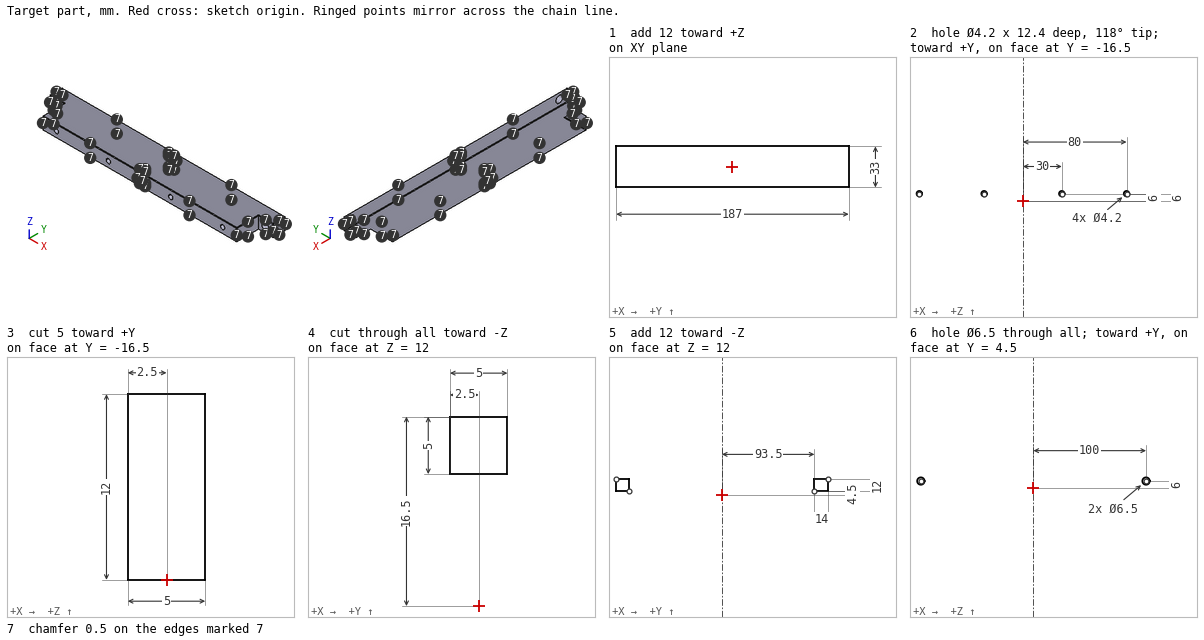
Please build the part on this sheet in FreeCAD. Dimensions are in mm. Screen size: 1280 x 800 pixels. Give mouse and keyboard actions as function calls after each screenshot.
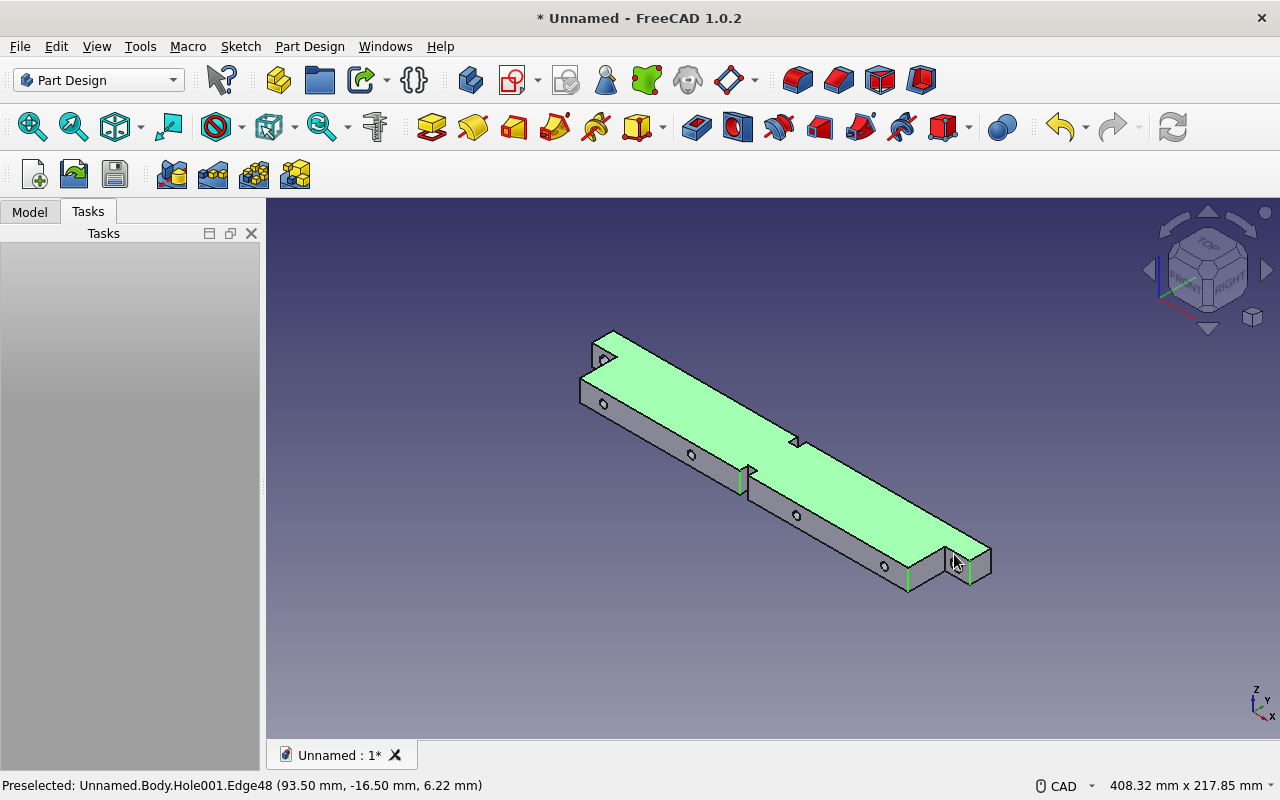
key(2)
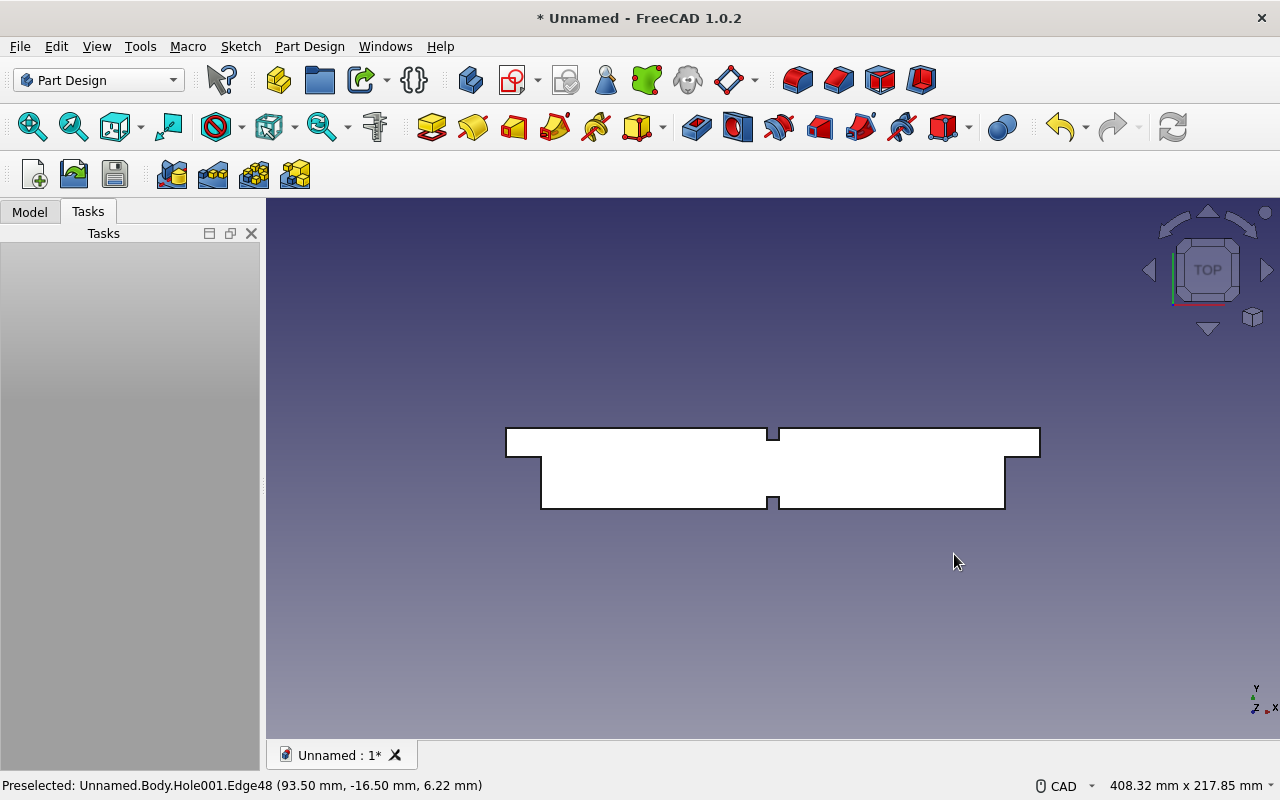
key(1)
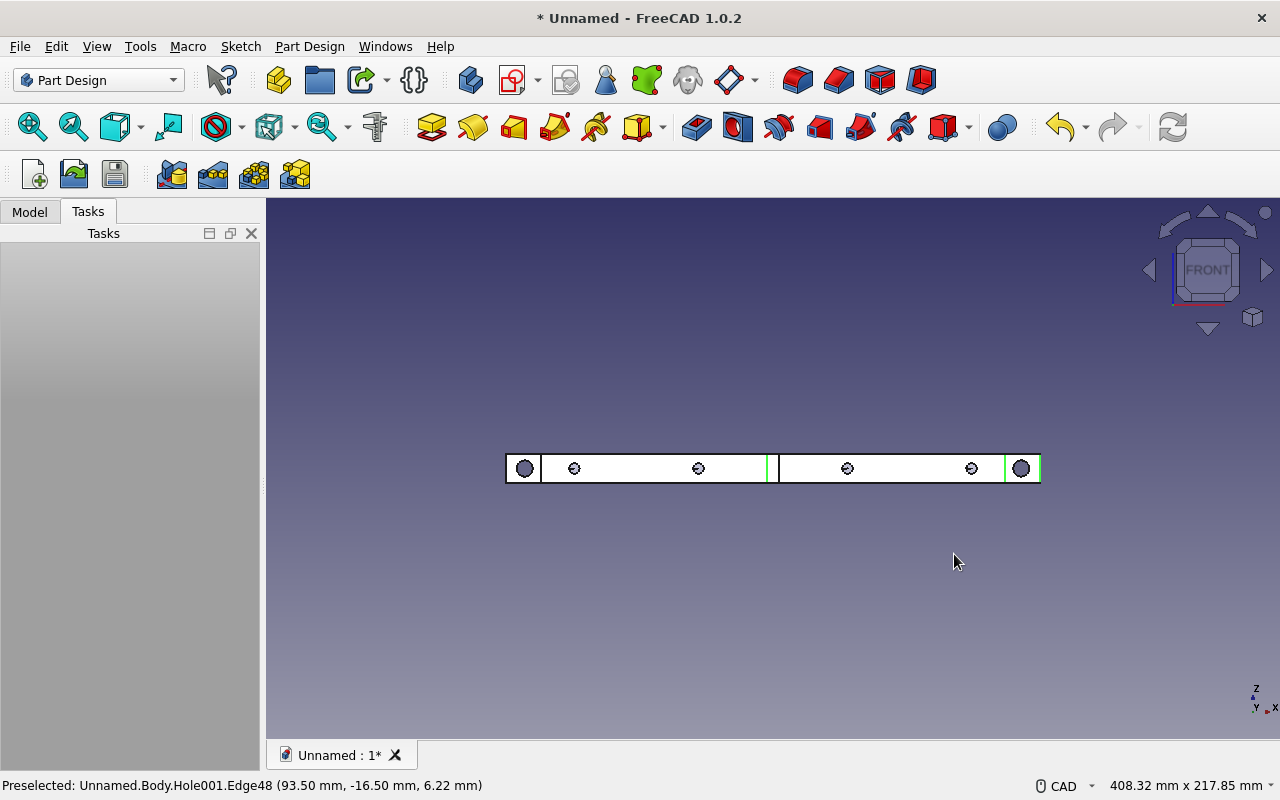
click(779, 467, ctrl)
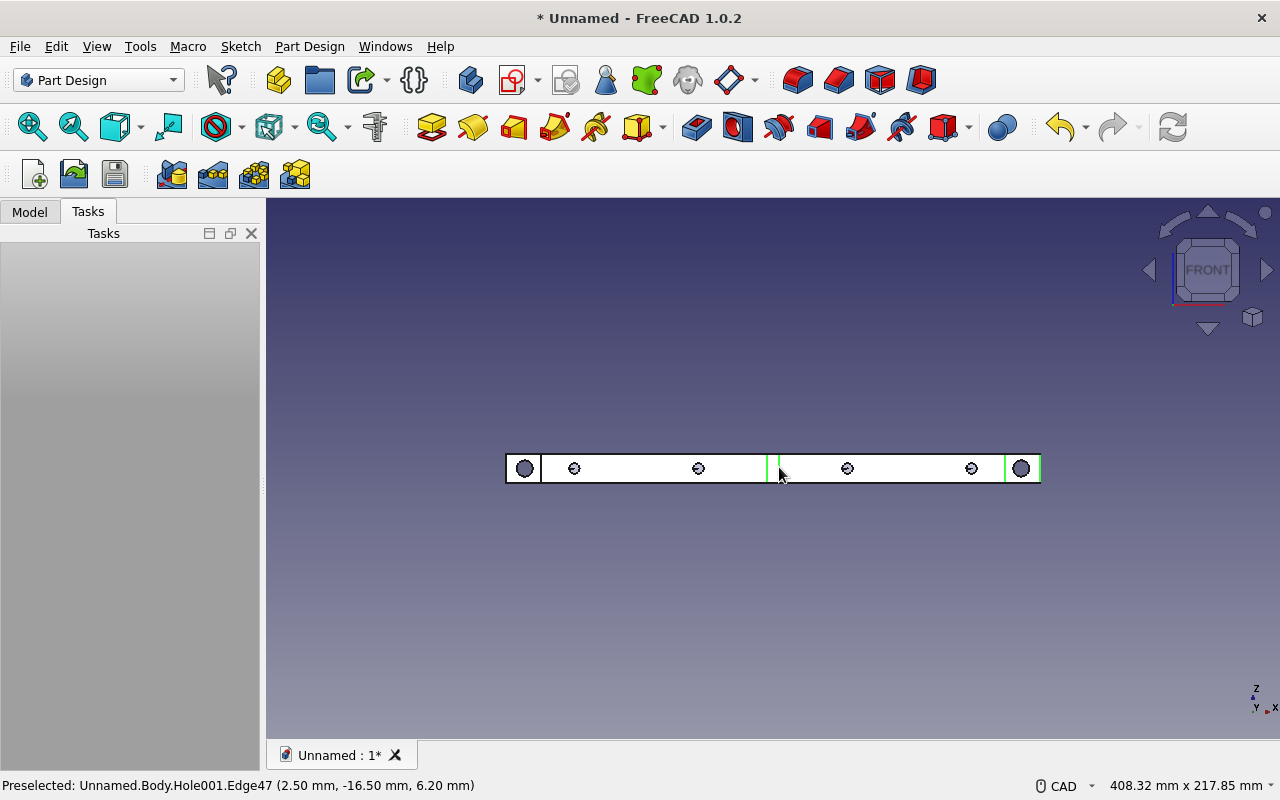
click(541, 467, ctrl)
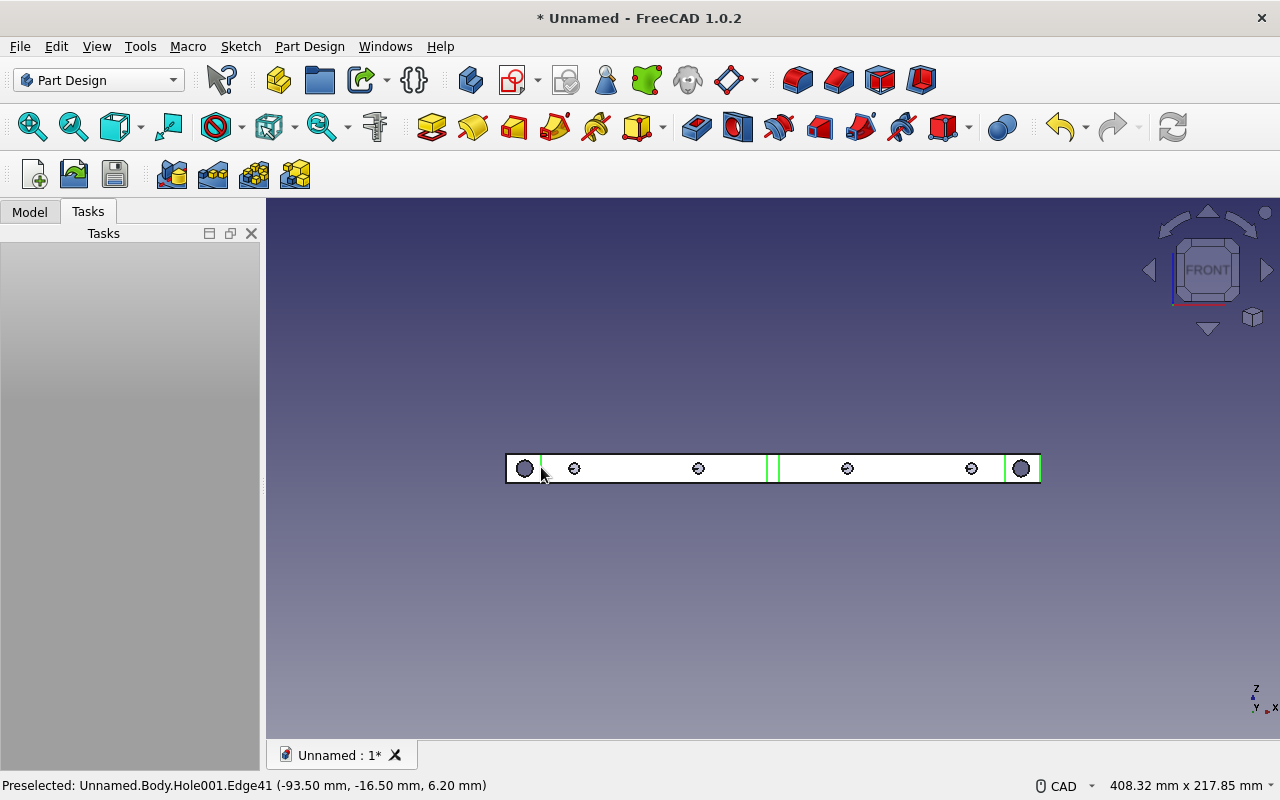
click(506, 467, ctrl)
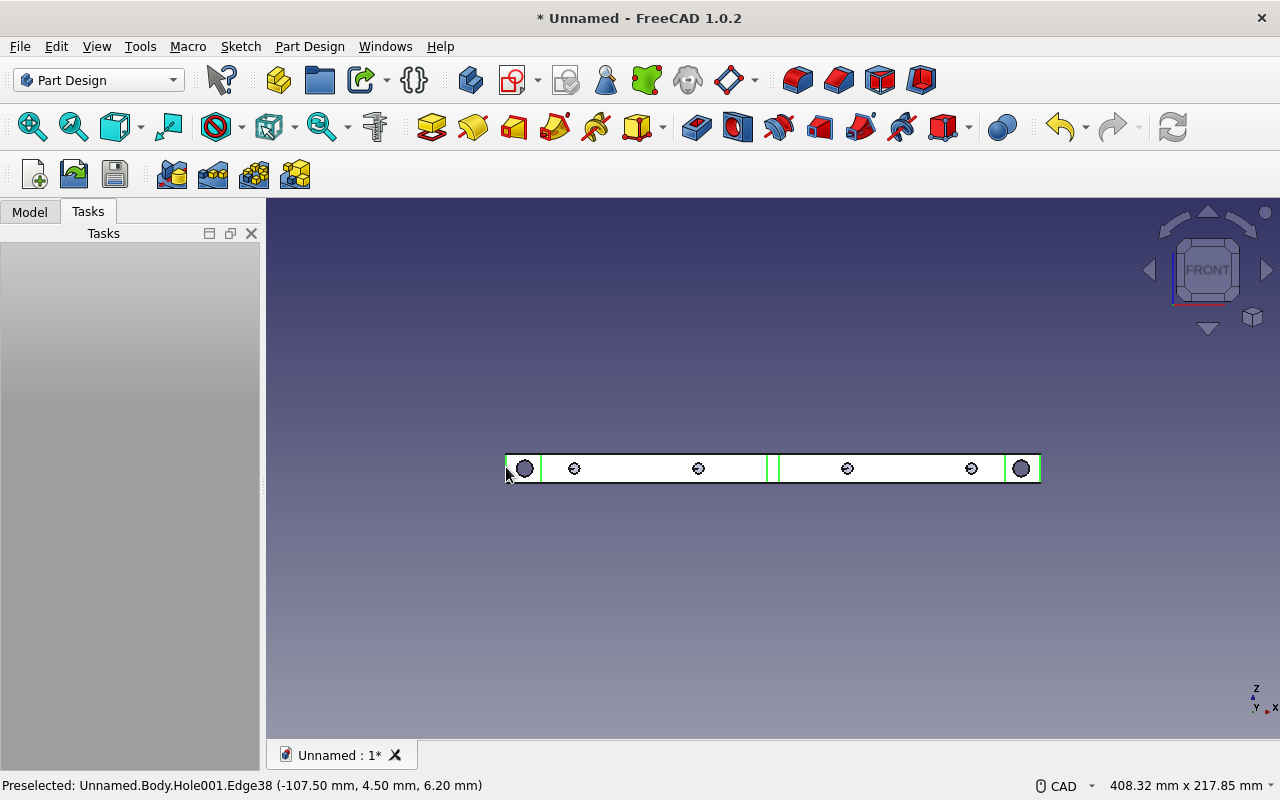
key(3)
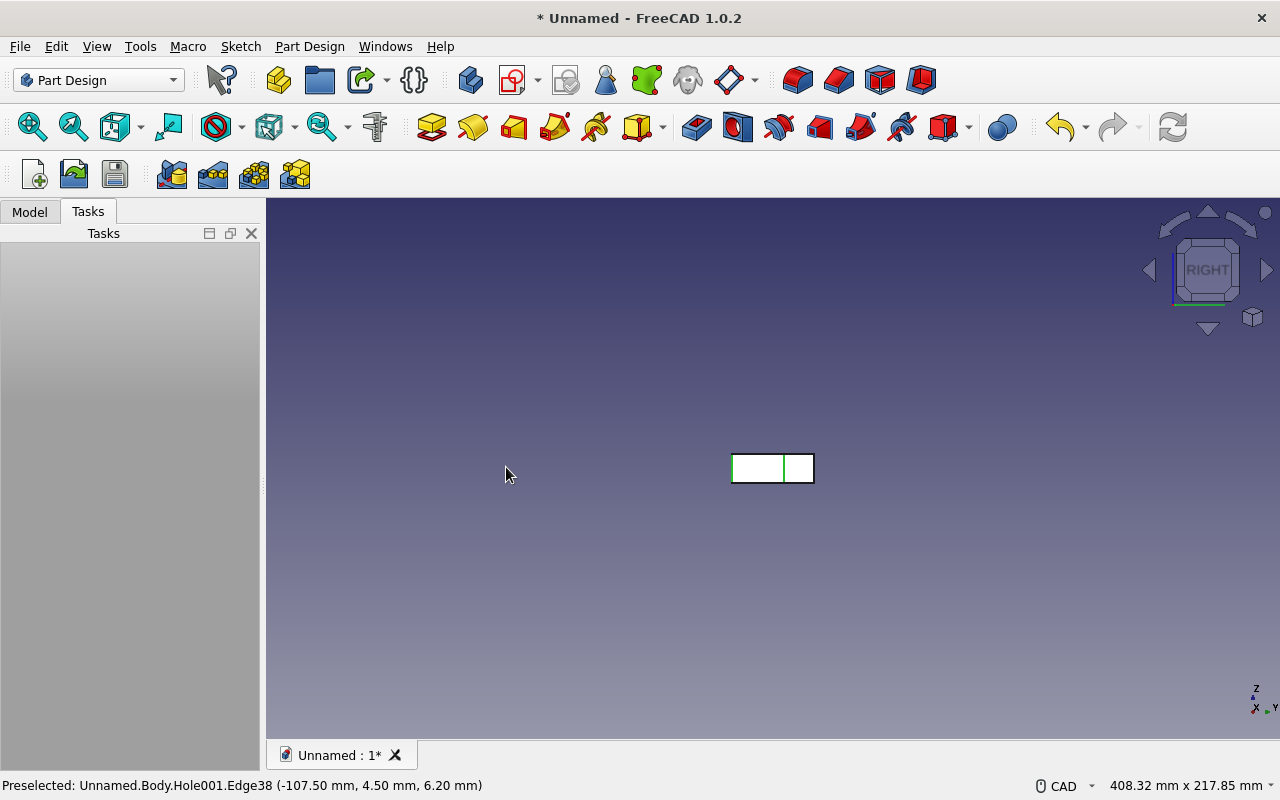
click(33, 128)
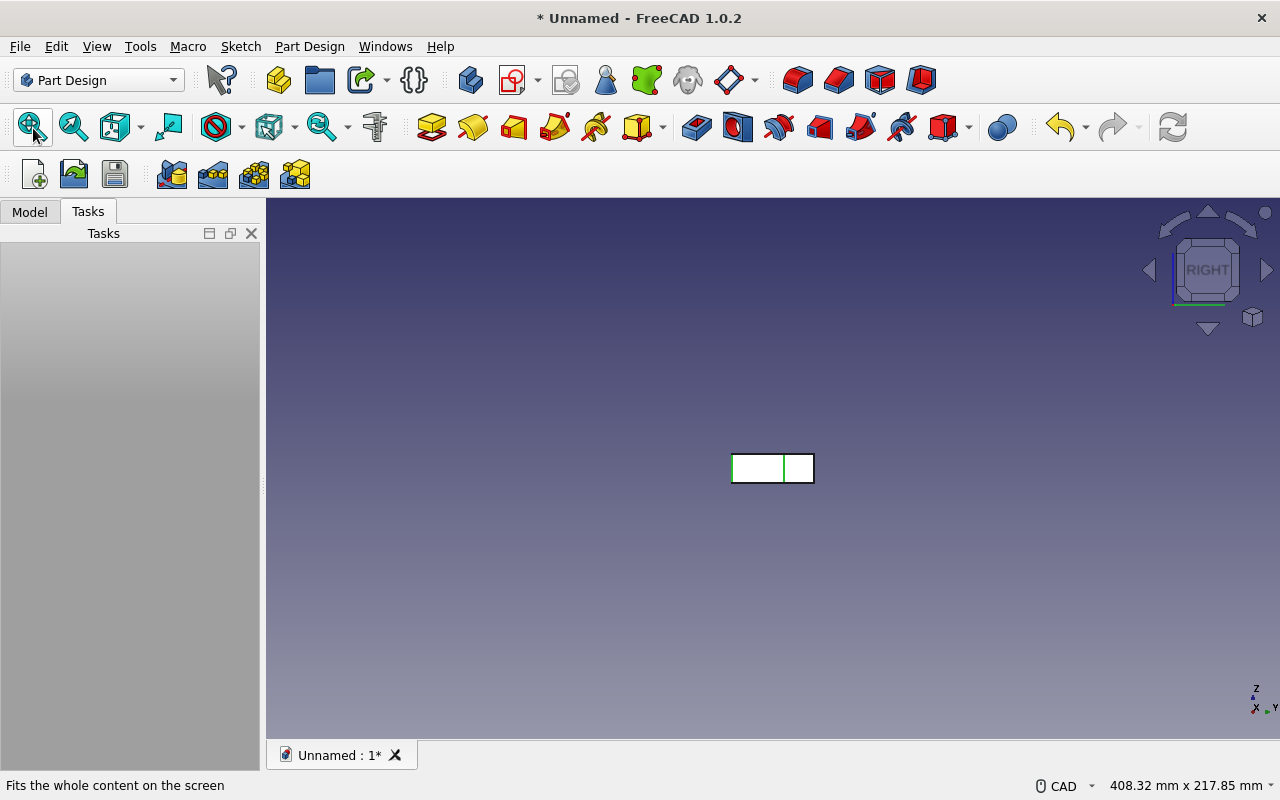
click(814, 467, ctrl)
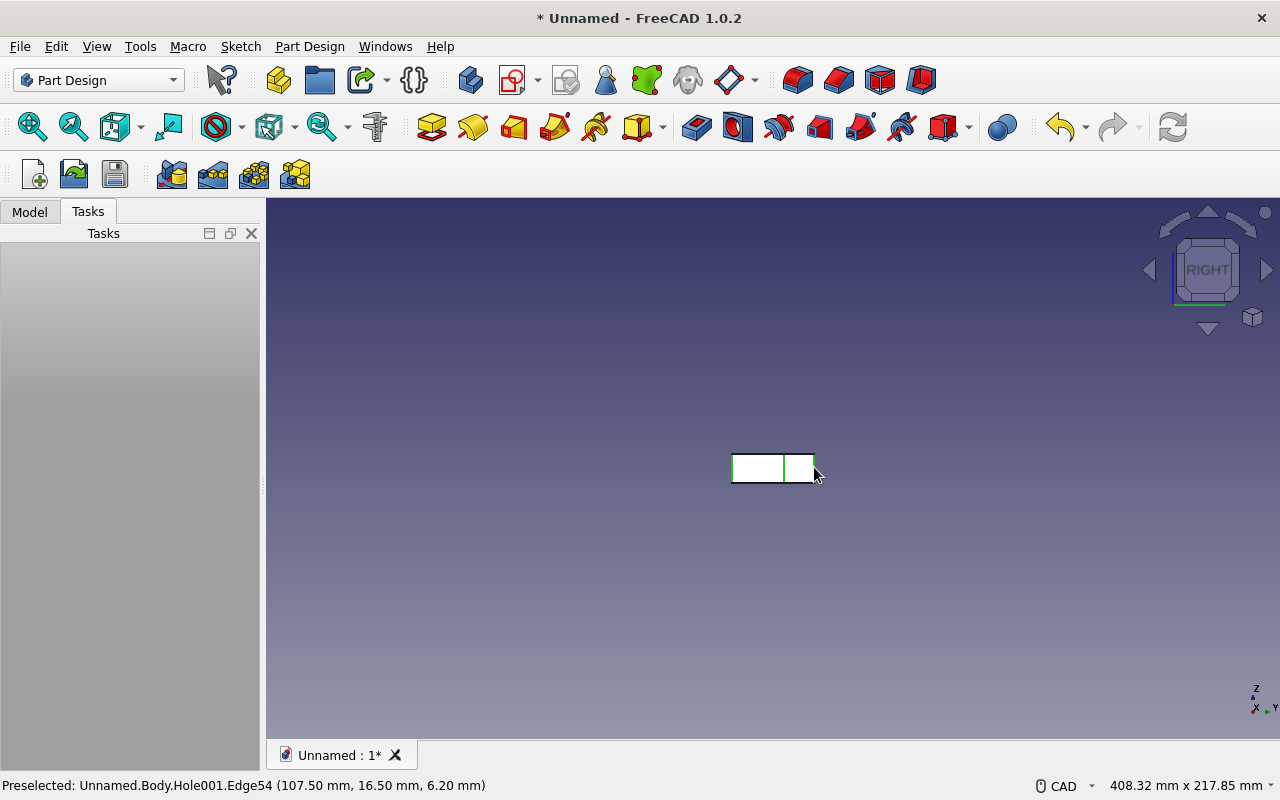
key(5)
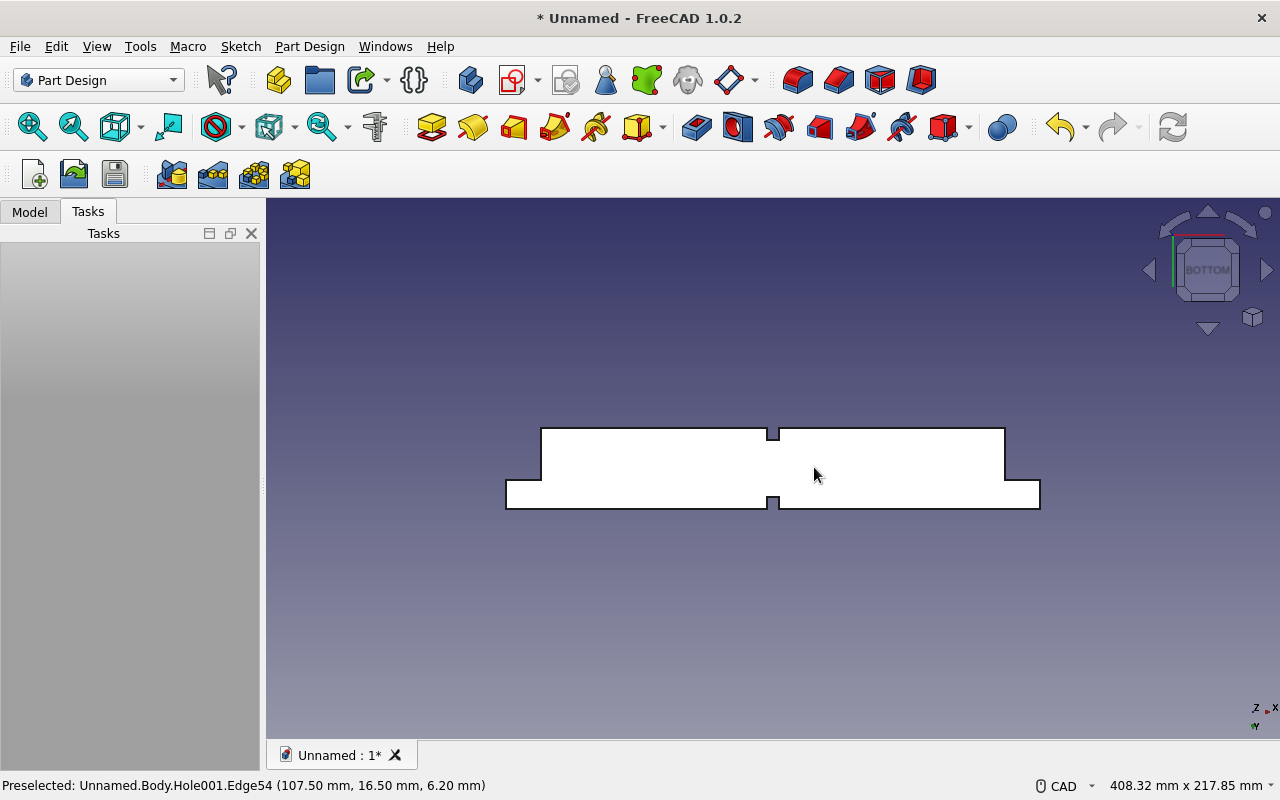
click(926, 467, ctrl)